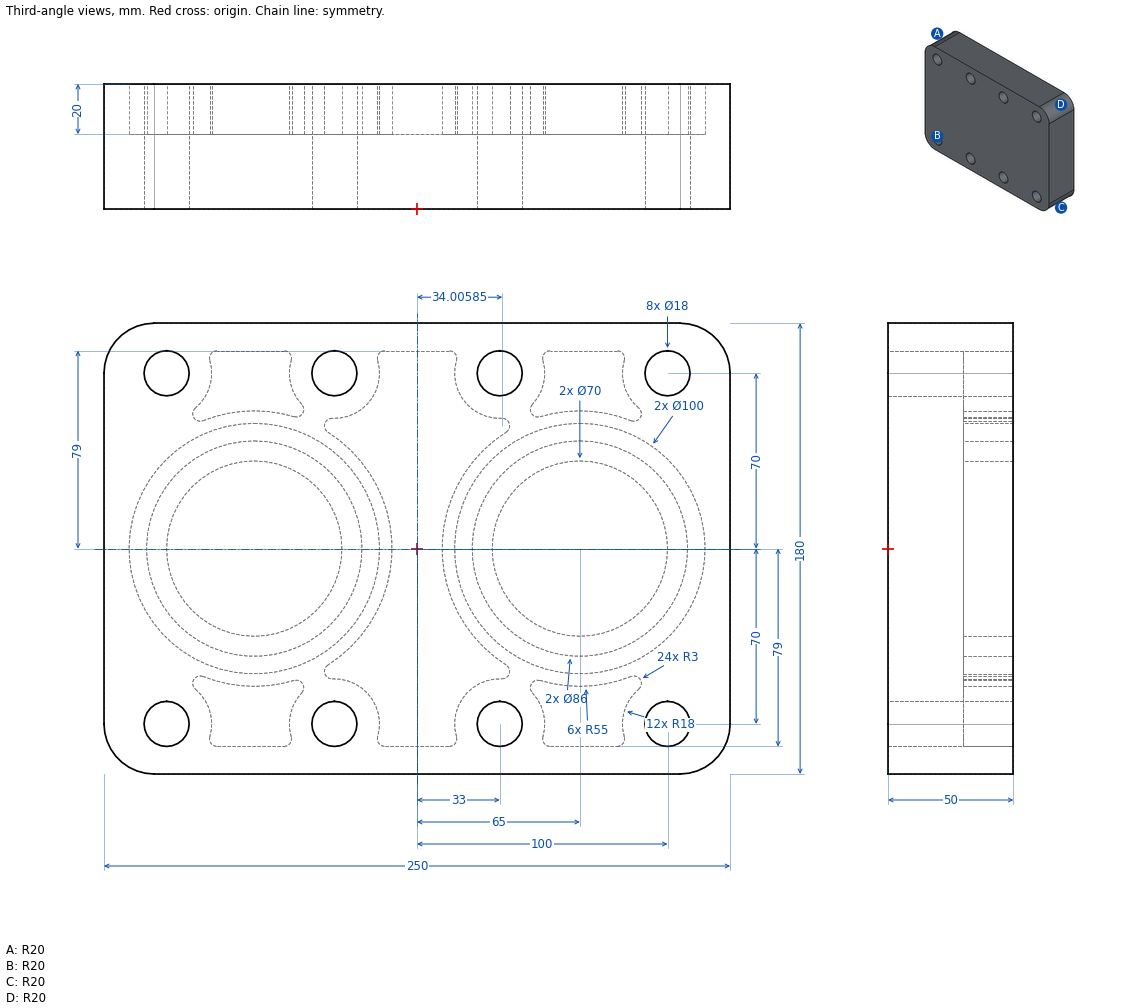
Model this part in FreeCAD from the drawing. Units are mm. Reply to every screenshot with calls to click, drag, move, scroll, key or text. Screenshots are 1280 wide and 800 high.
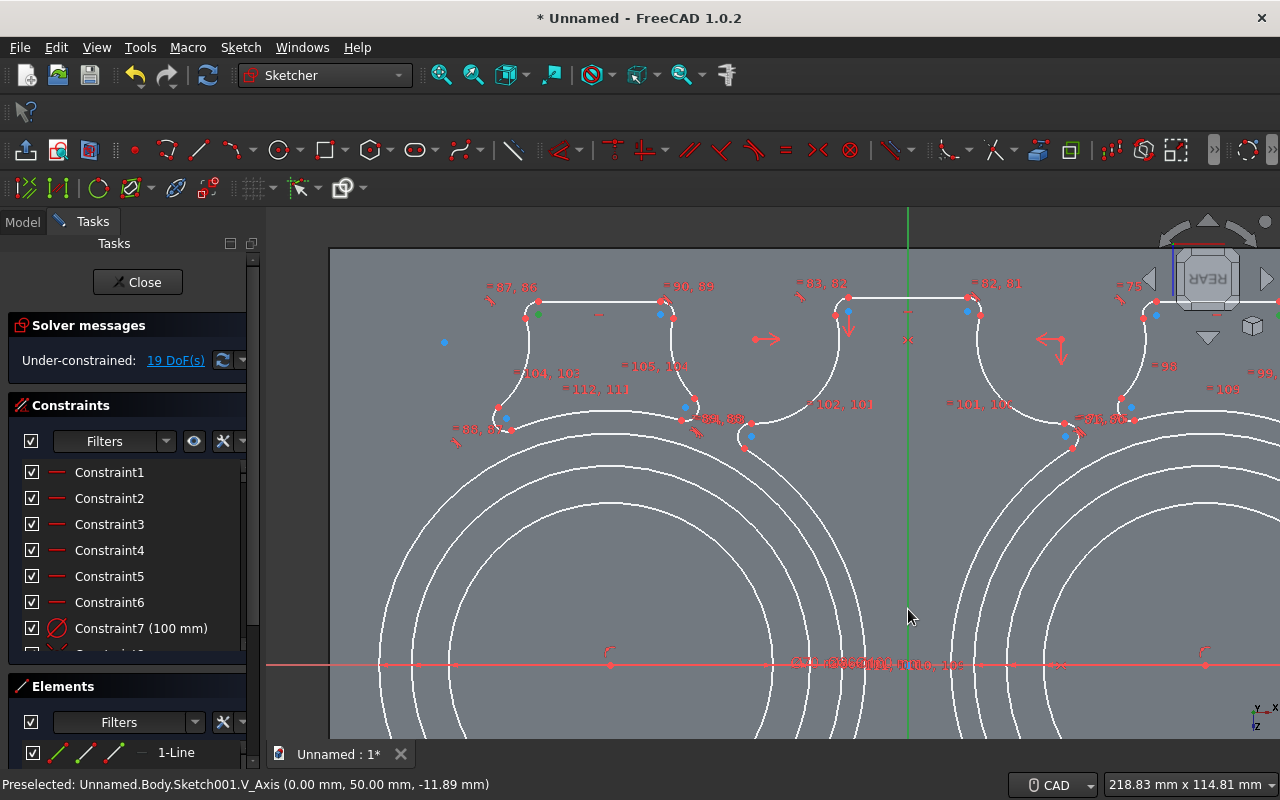
click(818, 150)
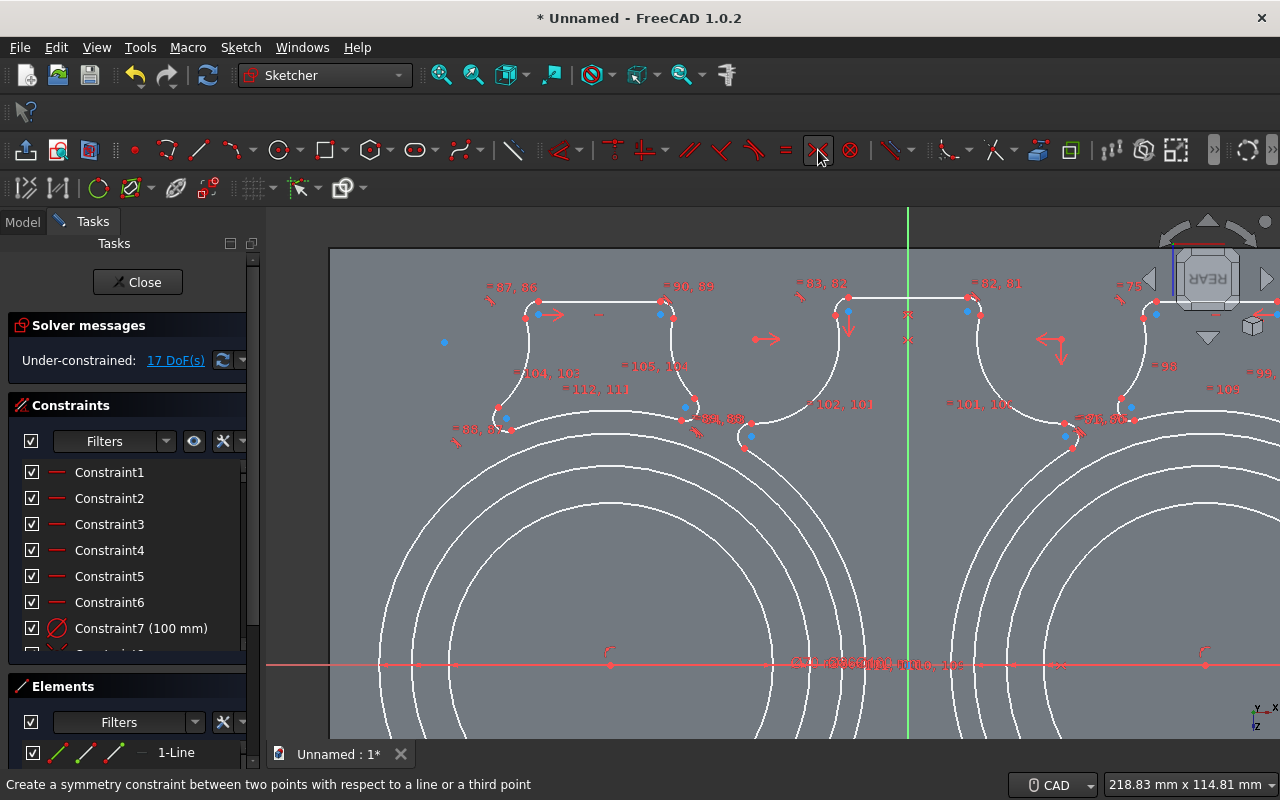
click(445, 343)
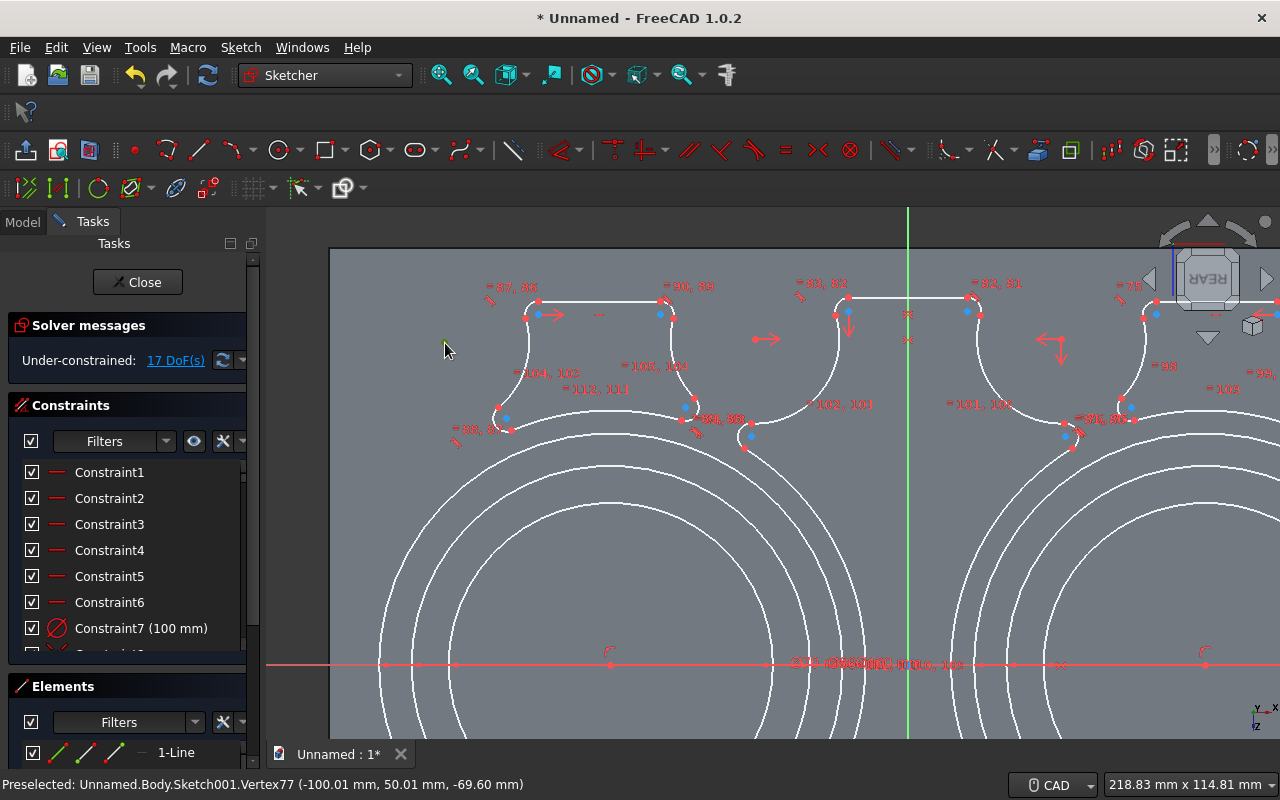
scroll(538, 316, down, 4)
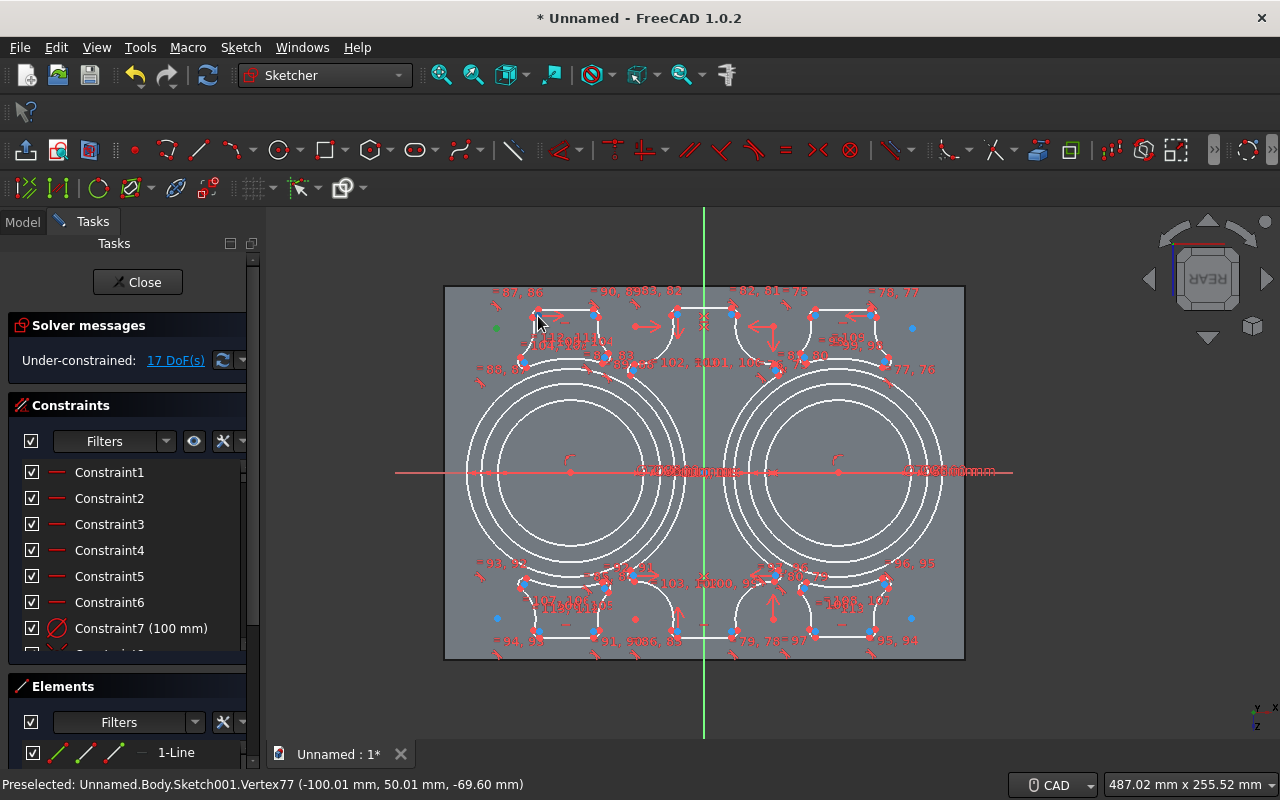
click(498, 619)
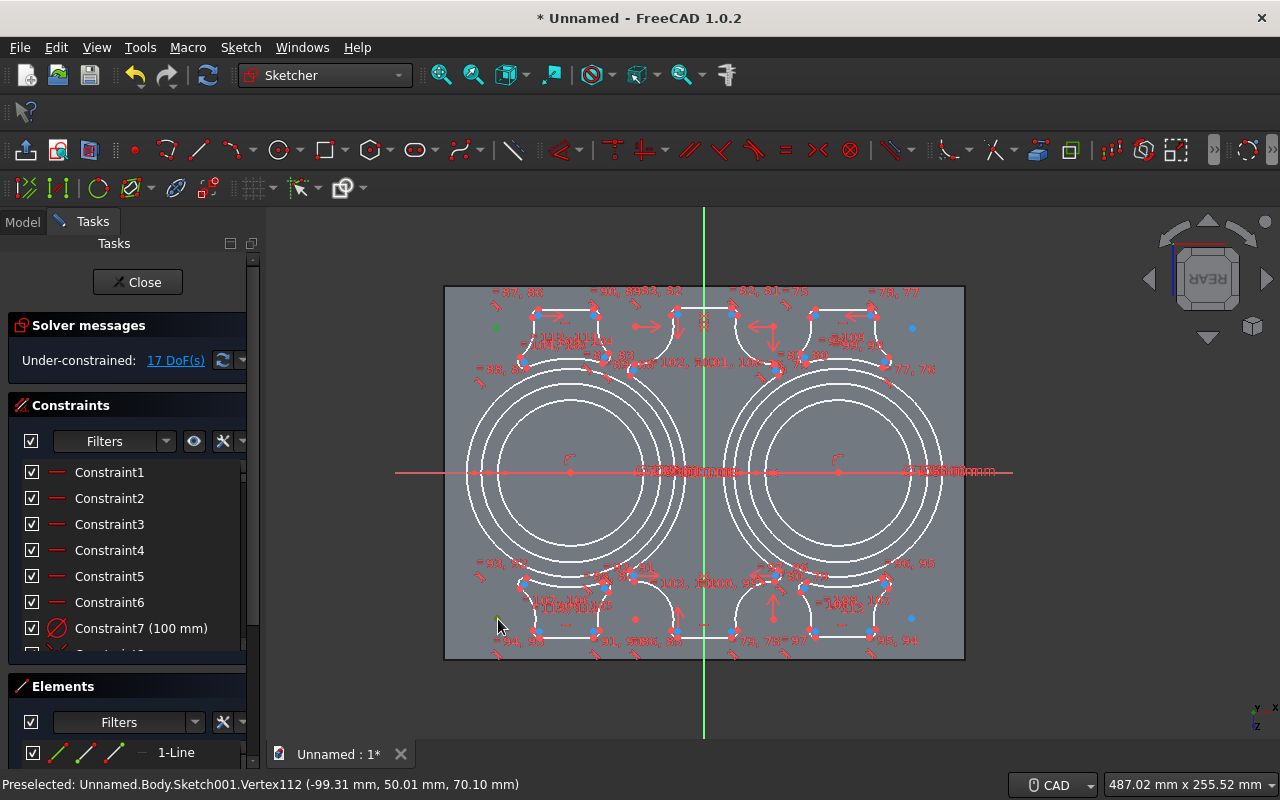
click(411, 473)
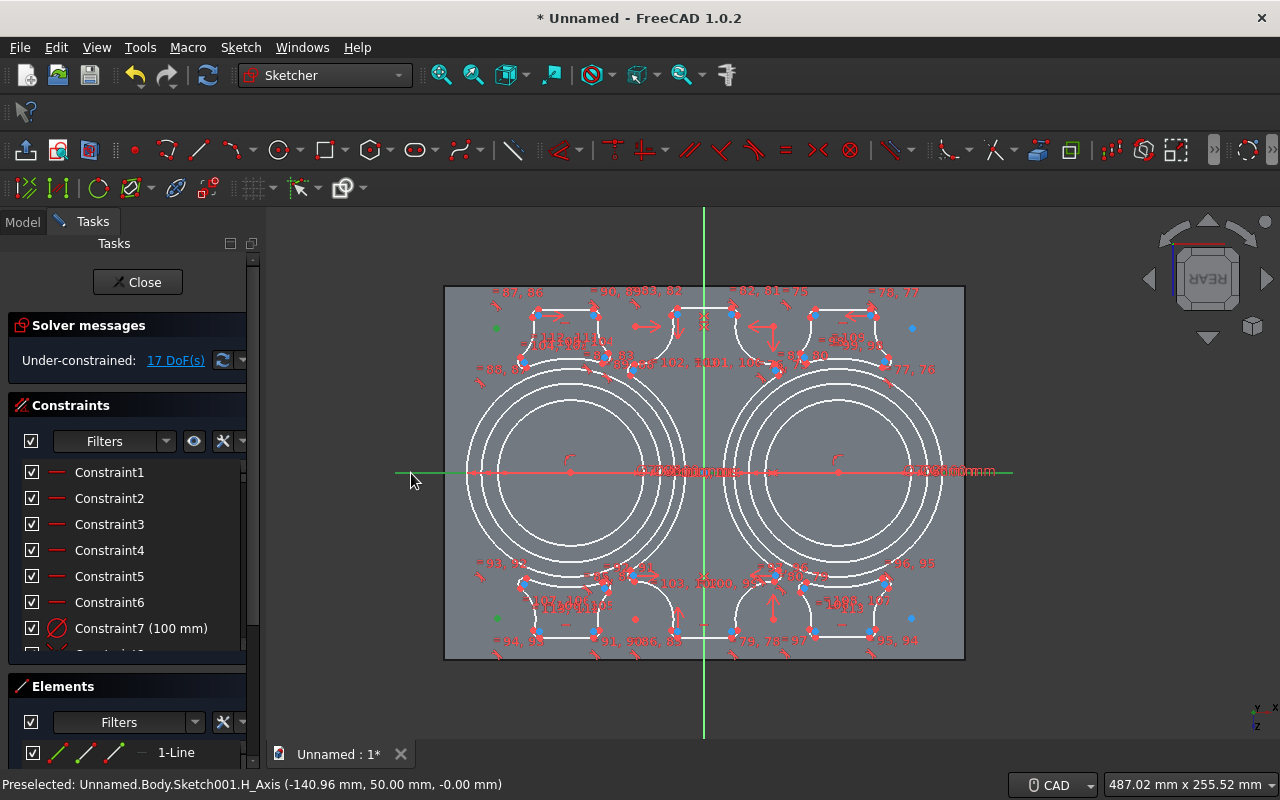
click(818, 150)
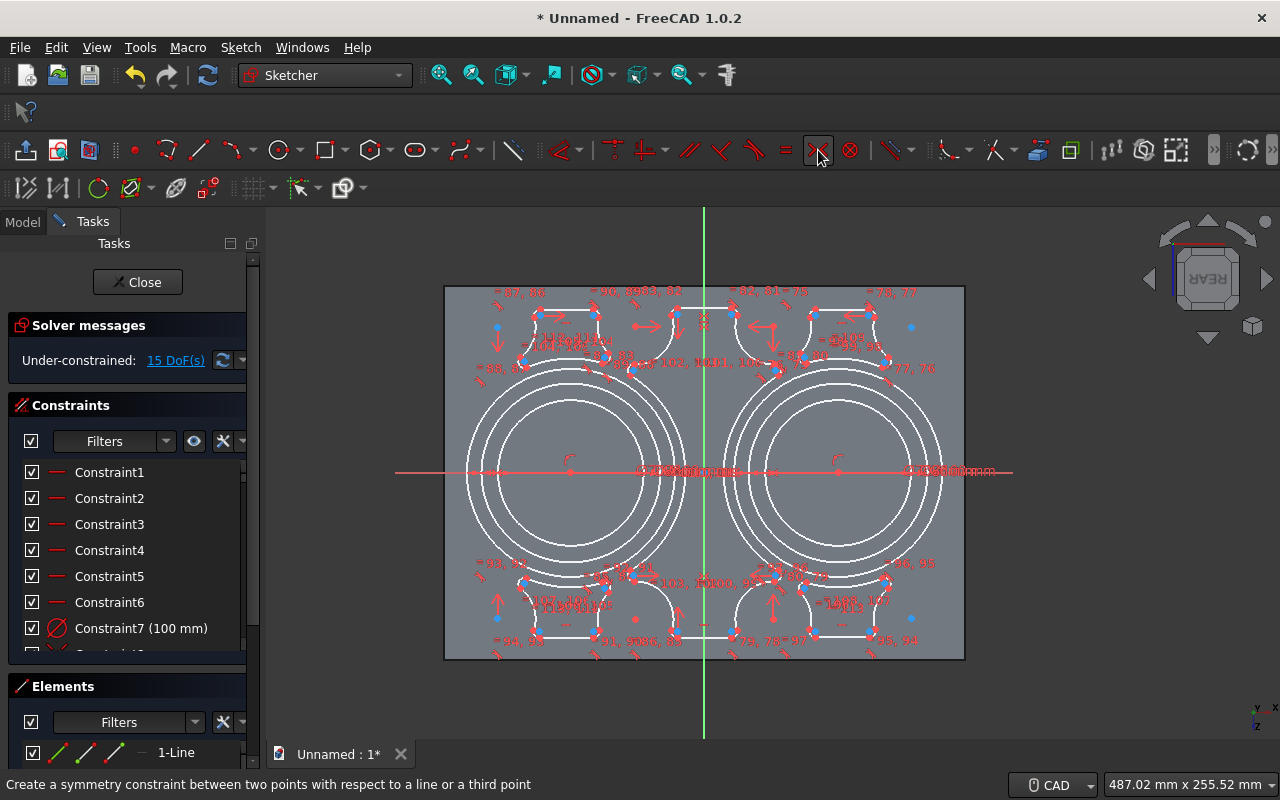
scroll(869, 316, up, 4)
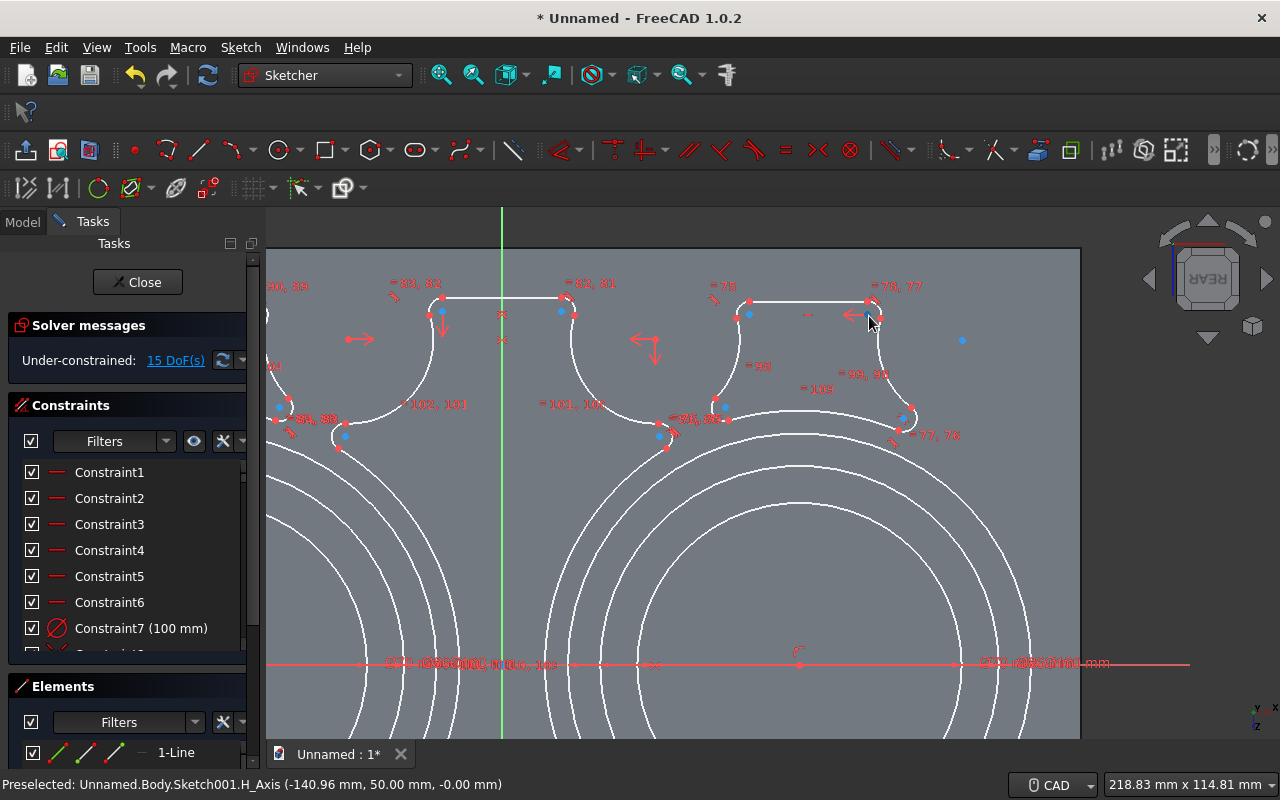
click(868, 315)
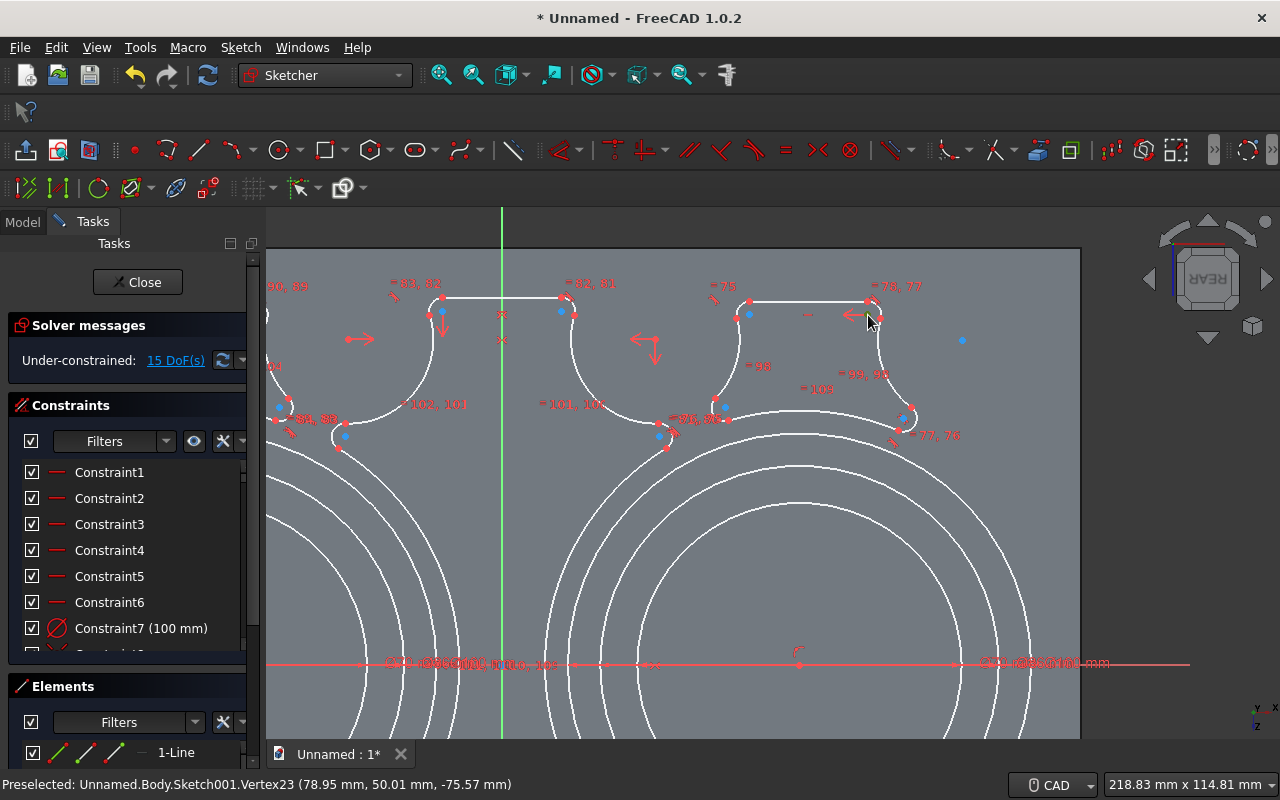
scroll(870, 316, down, 4)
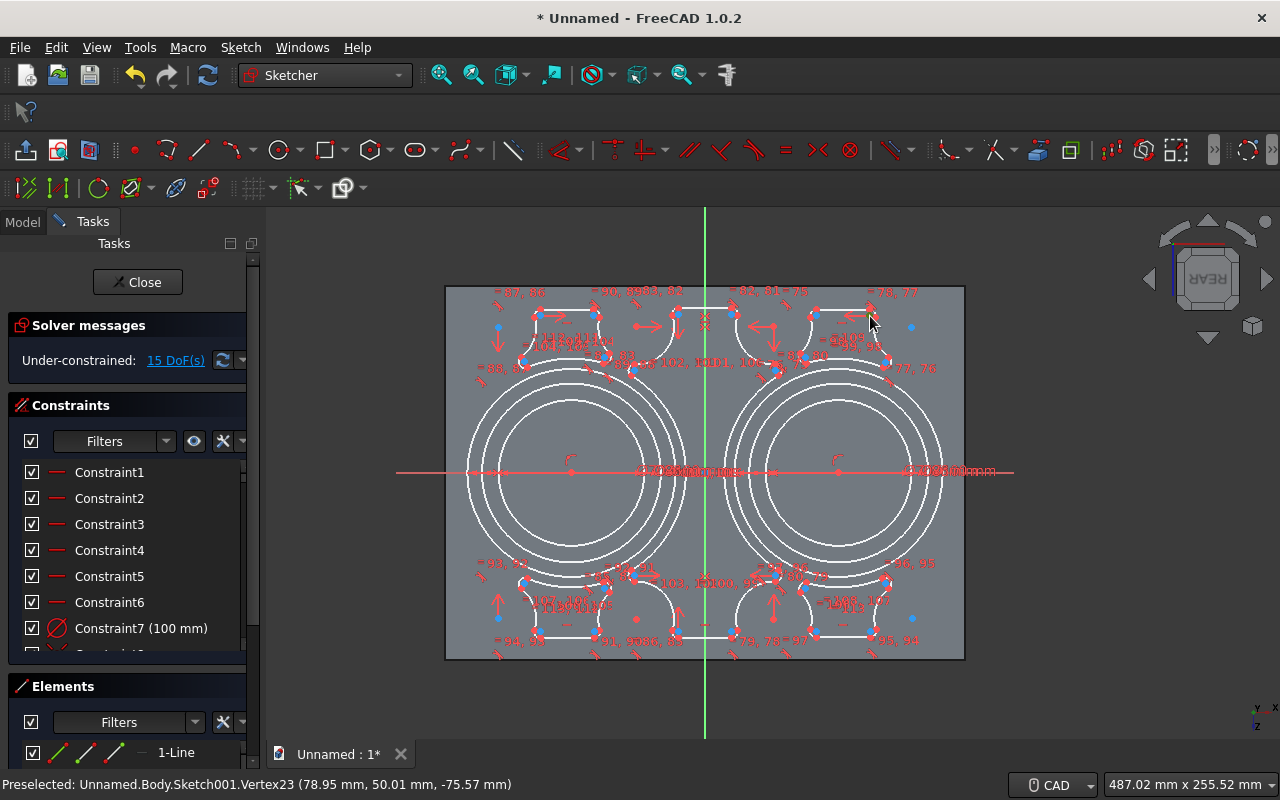
scroll(870, 631, up, 4)